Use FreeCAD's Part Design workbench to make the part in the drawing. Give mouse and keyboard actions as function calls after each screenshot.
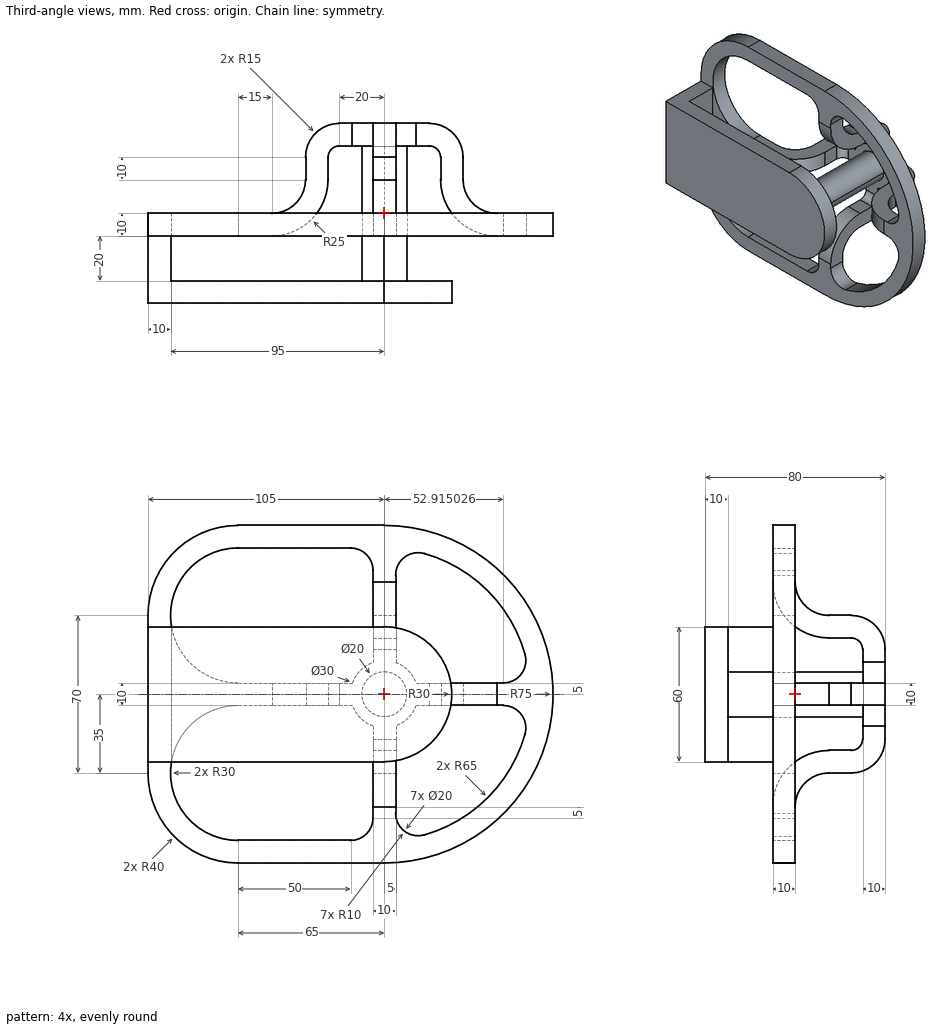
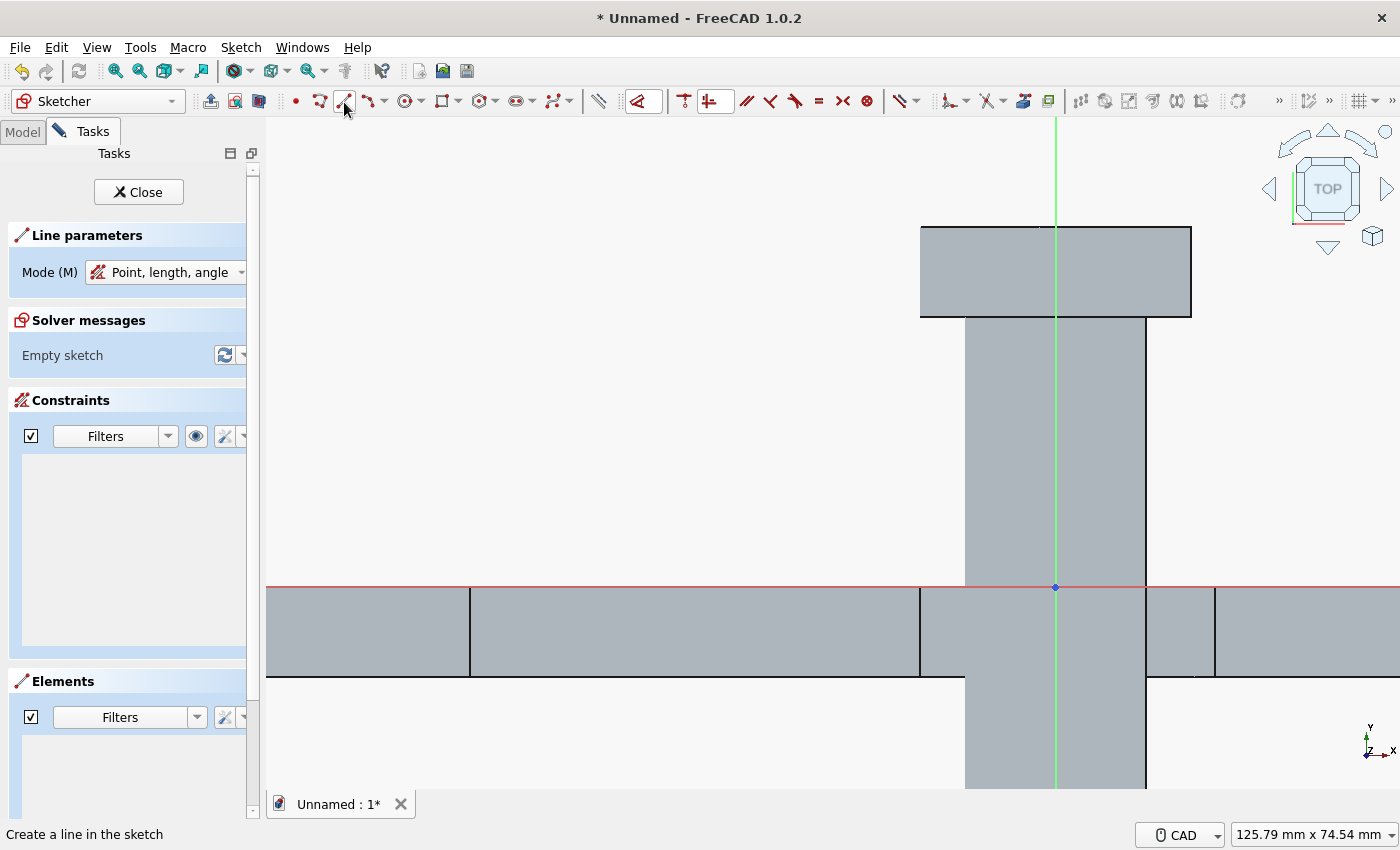
click(740, 362)
click(740, 452)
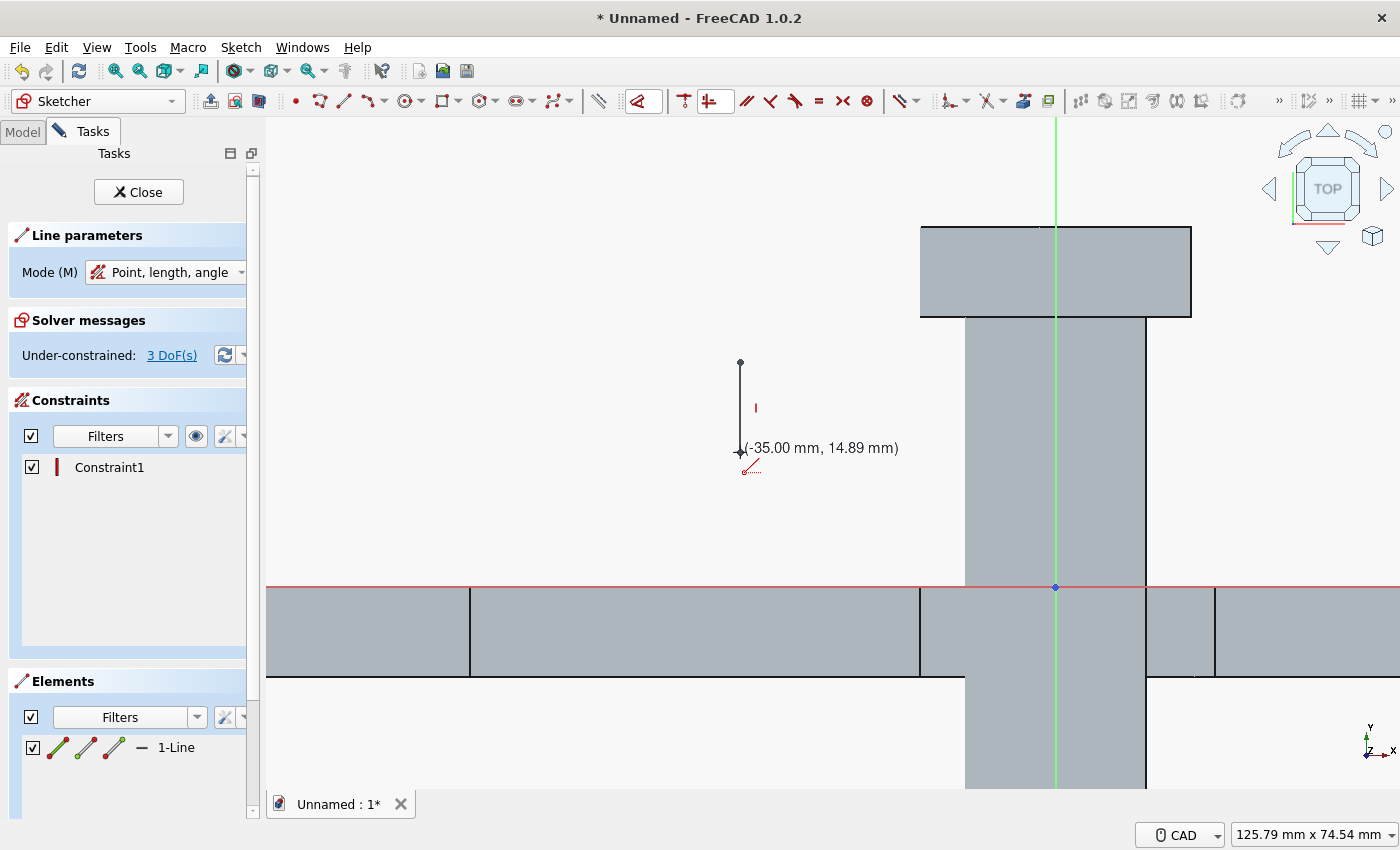
click(320, 102)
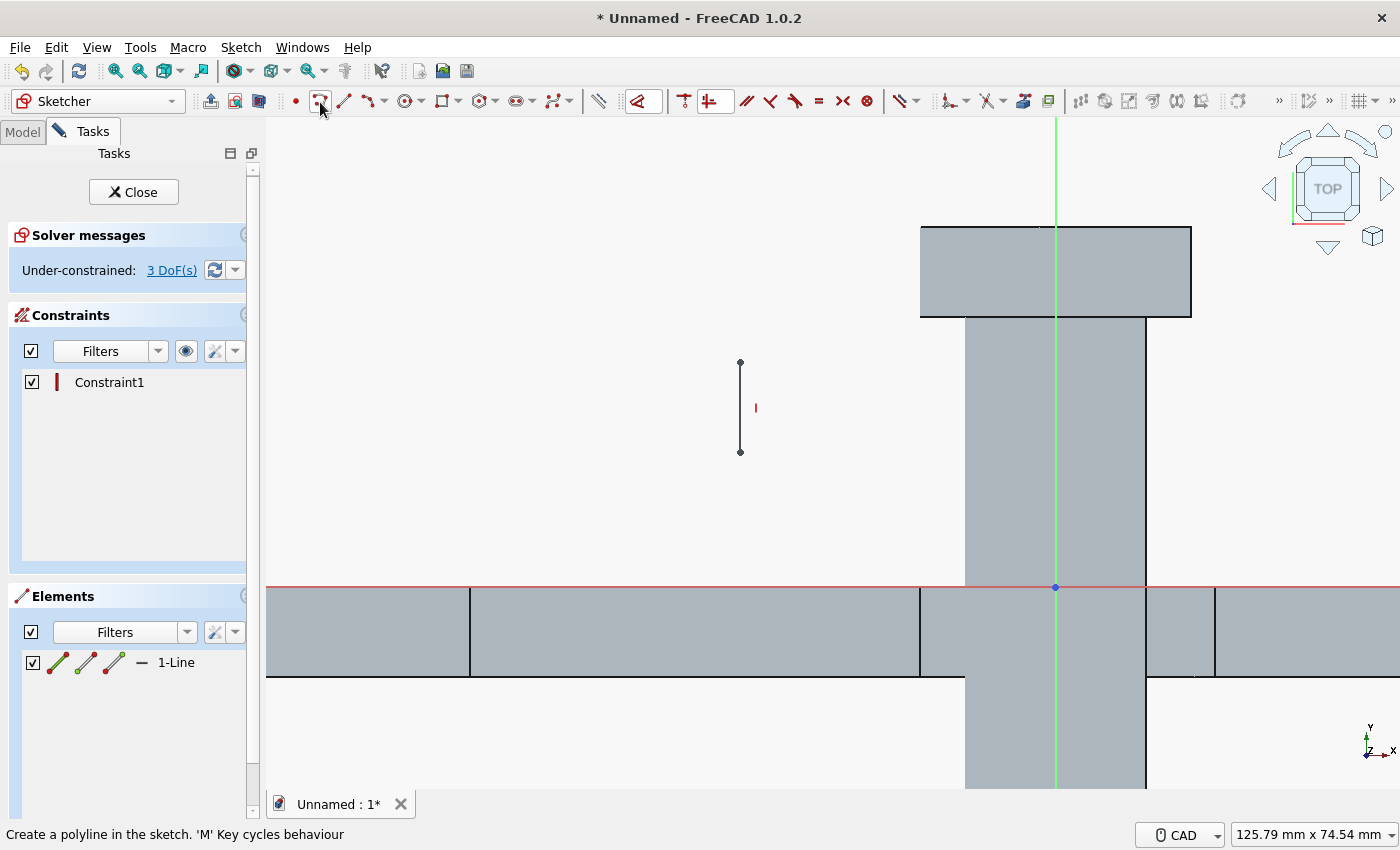
click(605, 587)
click(470, 578)
click(470, 677)
click(605, 677)
right_click(605, 677)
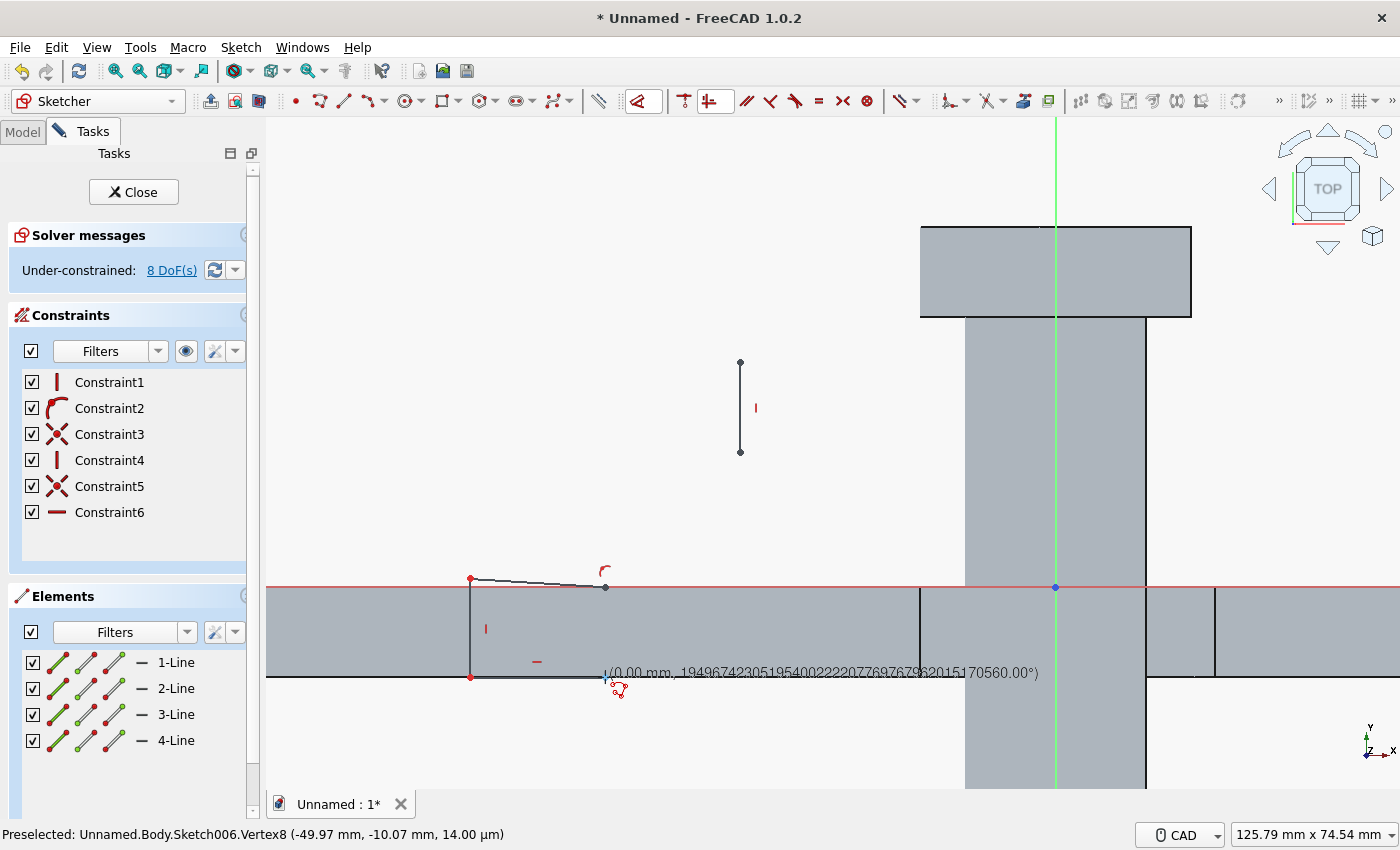
click(344, 102)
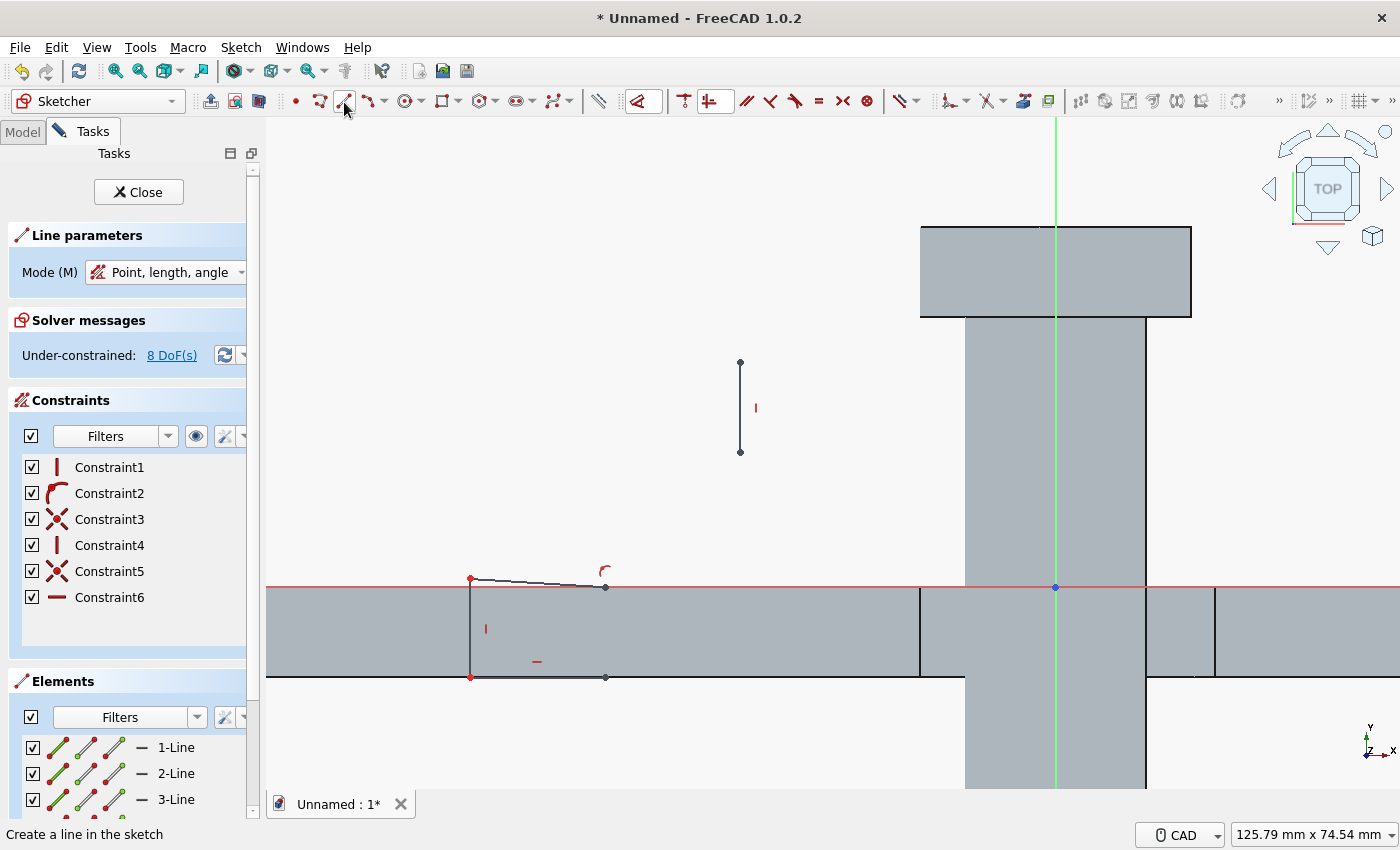
click(830, 452)
click(830, 362)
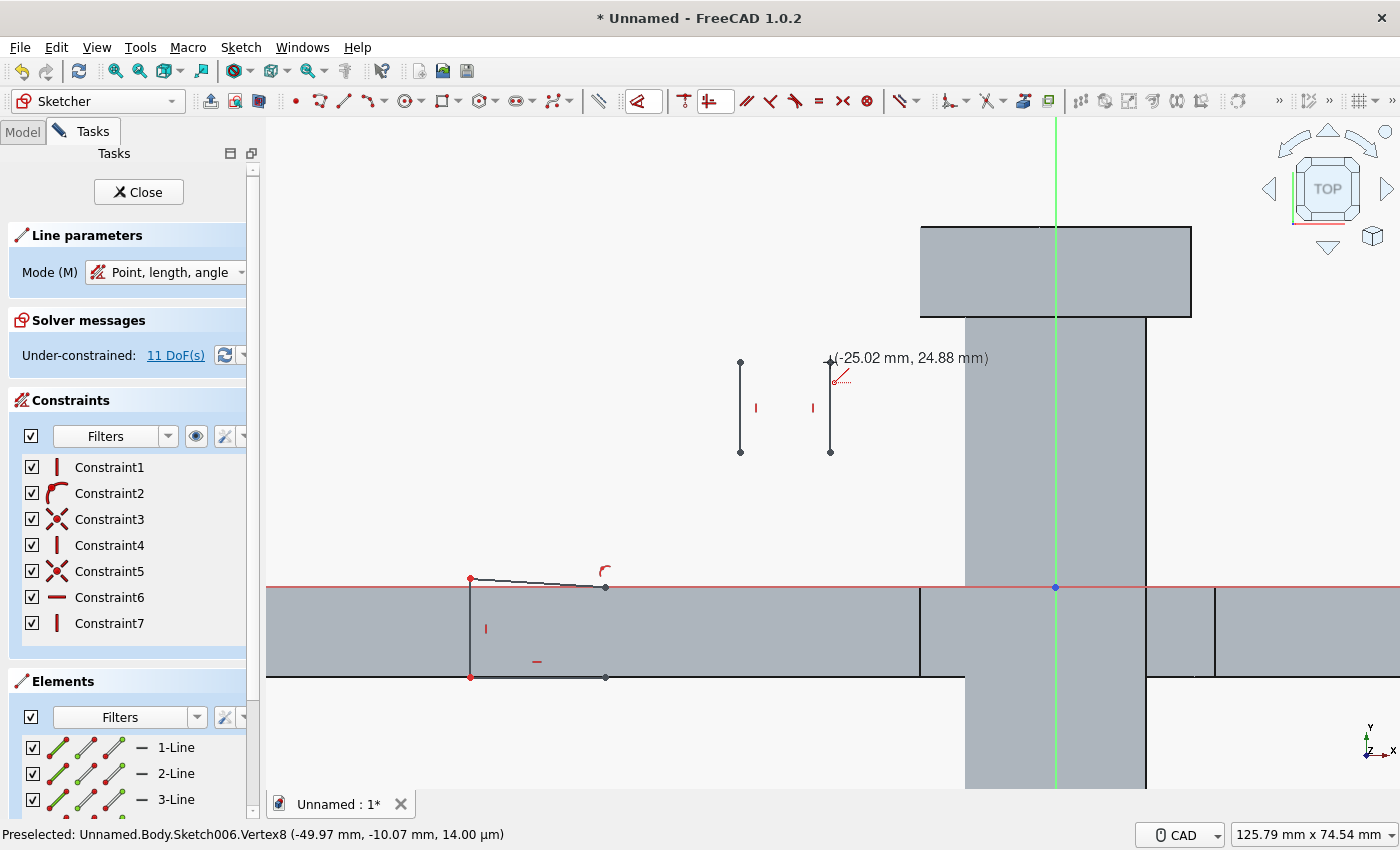
click(320, 102)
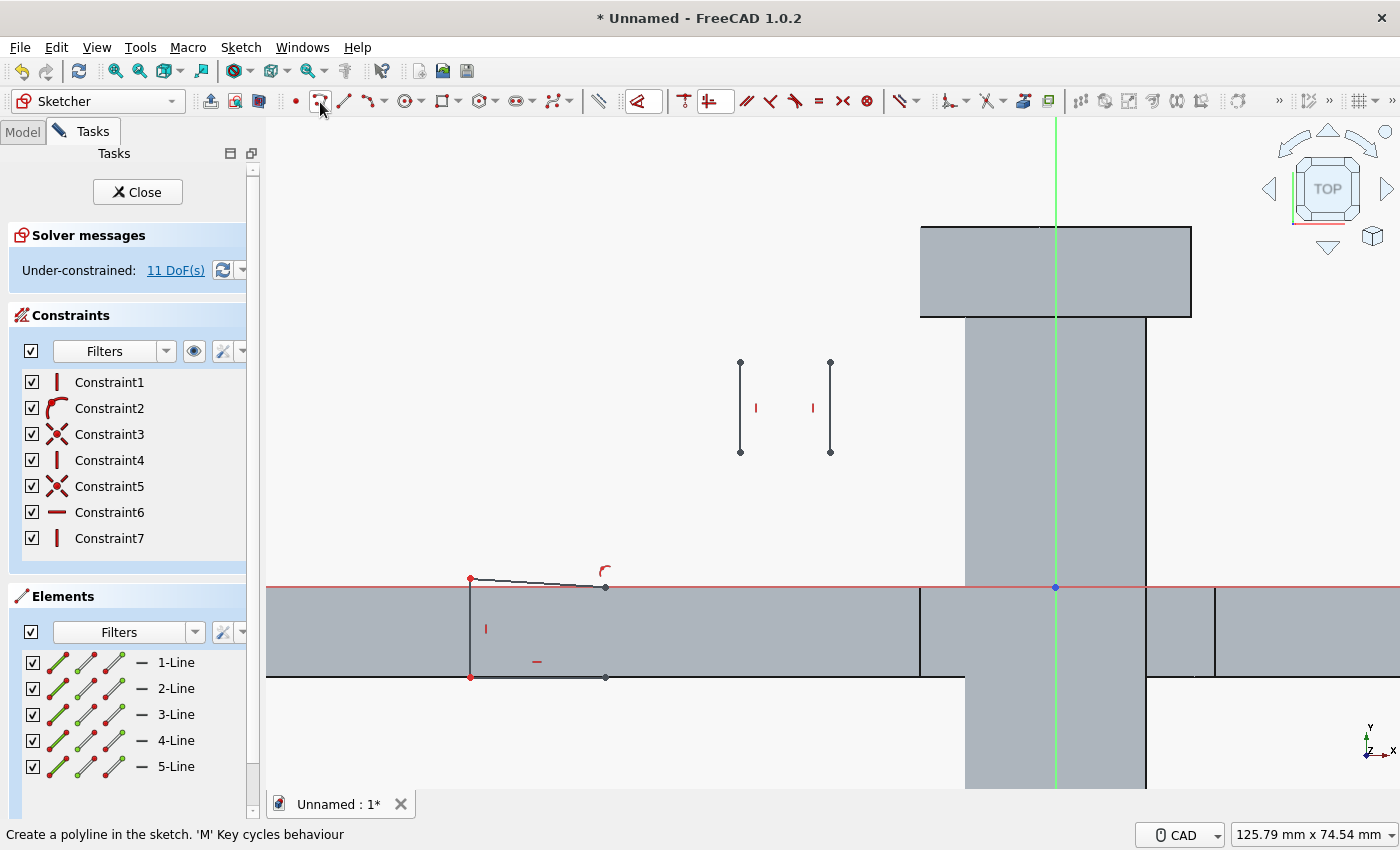
click(875, 317)
click(1056, 317)
click(1047, 227)
click(875, 227)
right_click(875, 227)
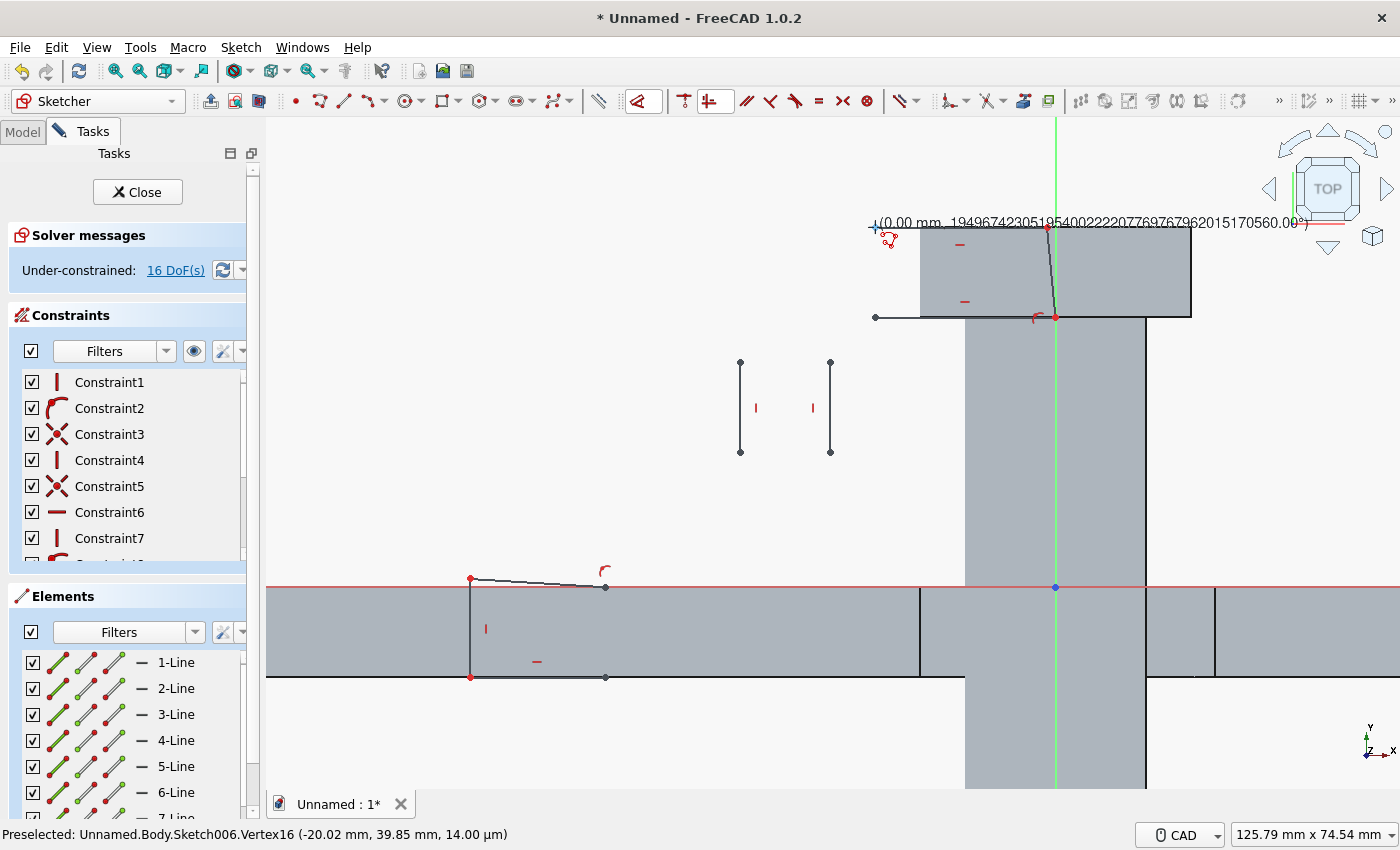
click(368, 102)